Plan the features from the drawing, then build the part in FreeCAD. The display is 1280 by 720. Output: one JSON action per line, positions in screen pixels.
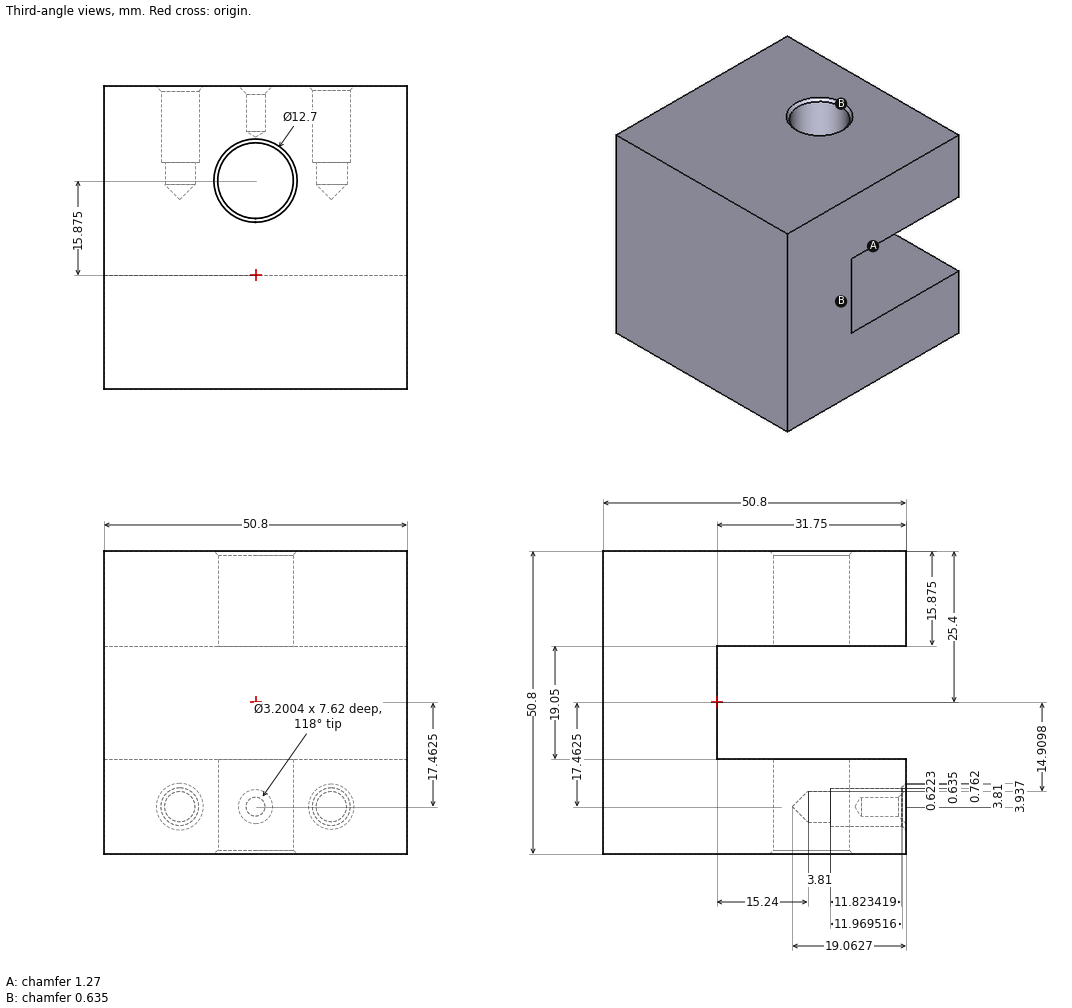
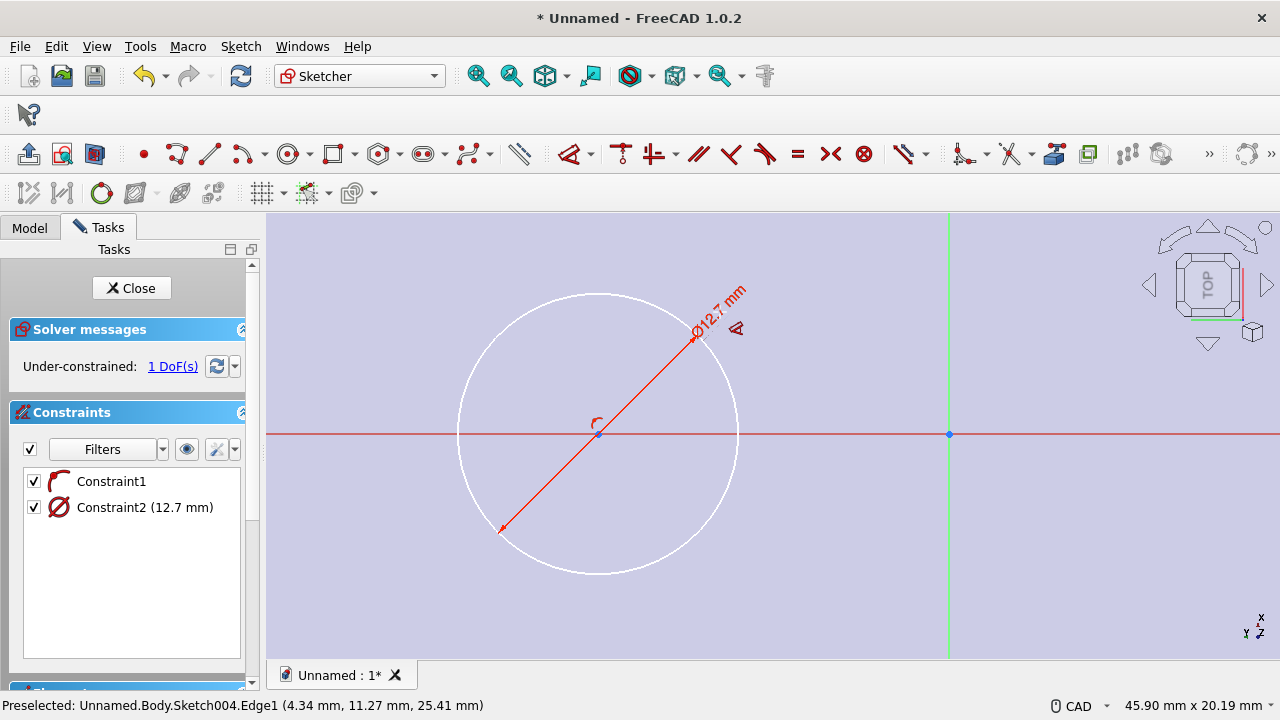
{"action": "left_click", "coordinate": [598, 434]}
{"action": "left_click", "coordinate": [774, 468]}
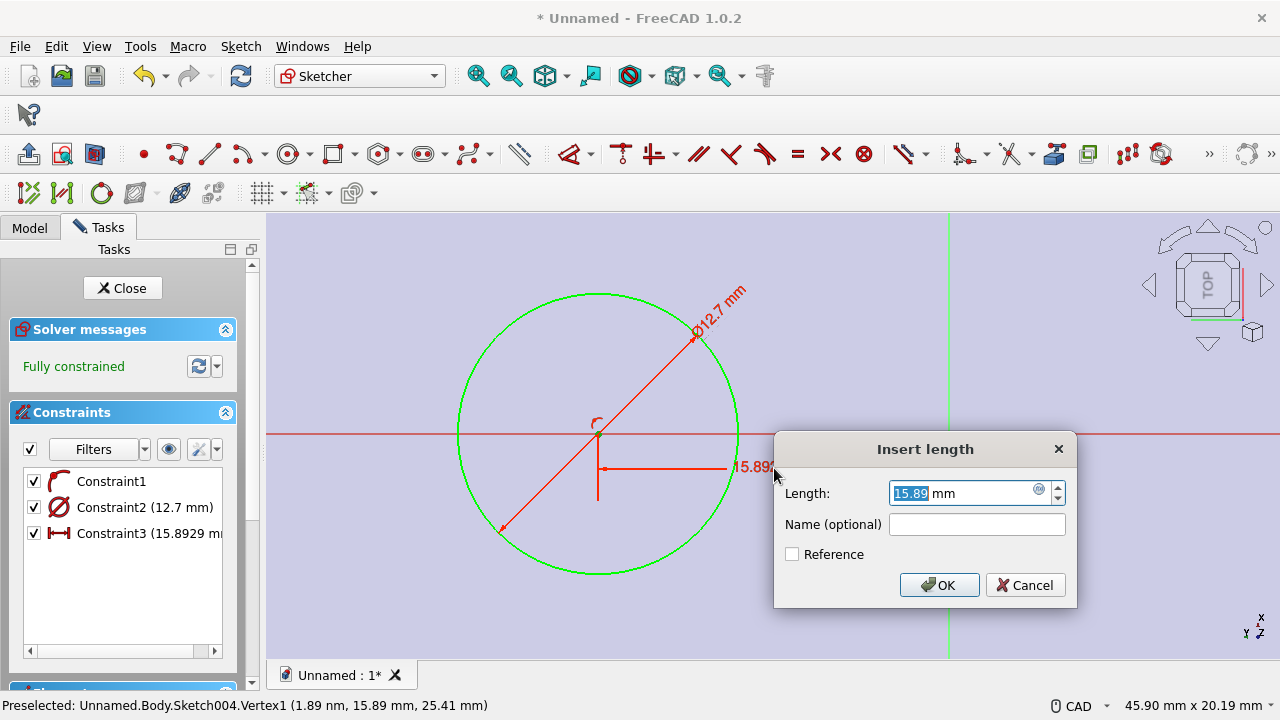
{"action": "type", "text": "15.875"}
{"action": "key", "text": "Return"}
{"action": "key", "text": "Escape"}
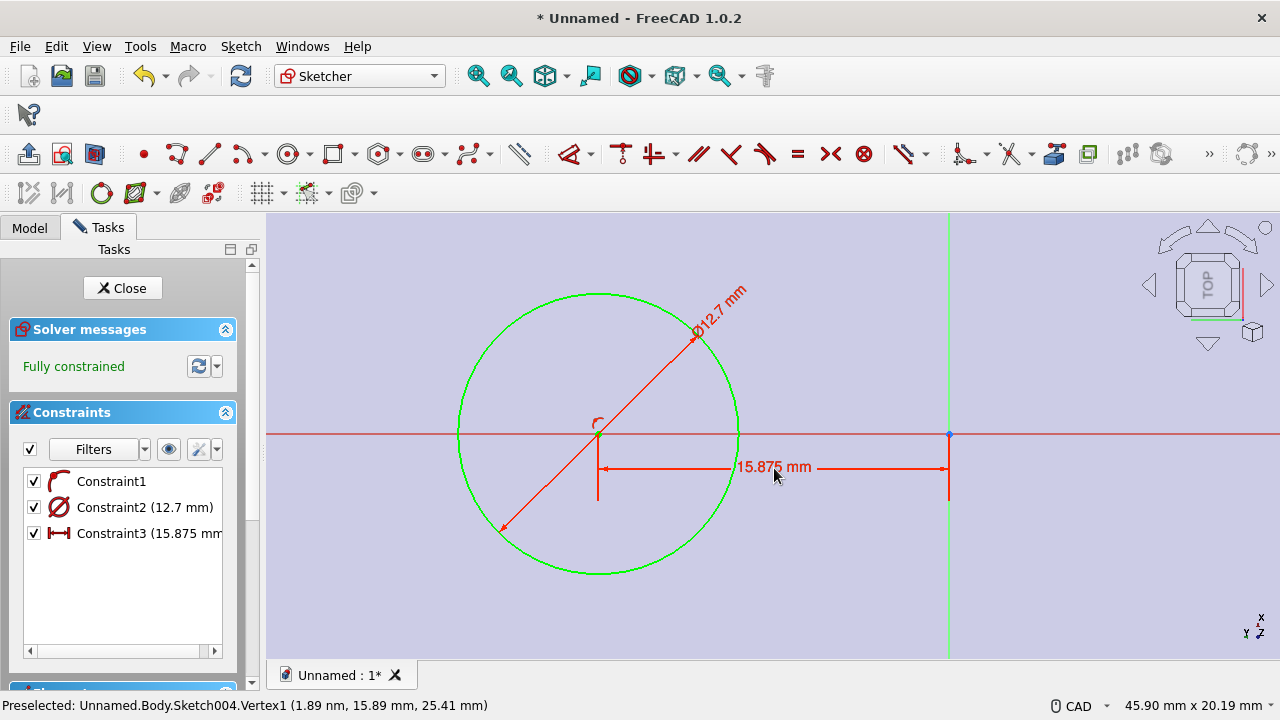
{"action": "left_click", "coordinate": [123, 288]}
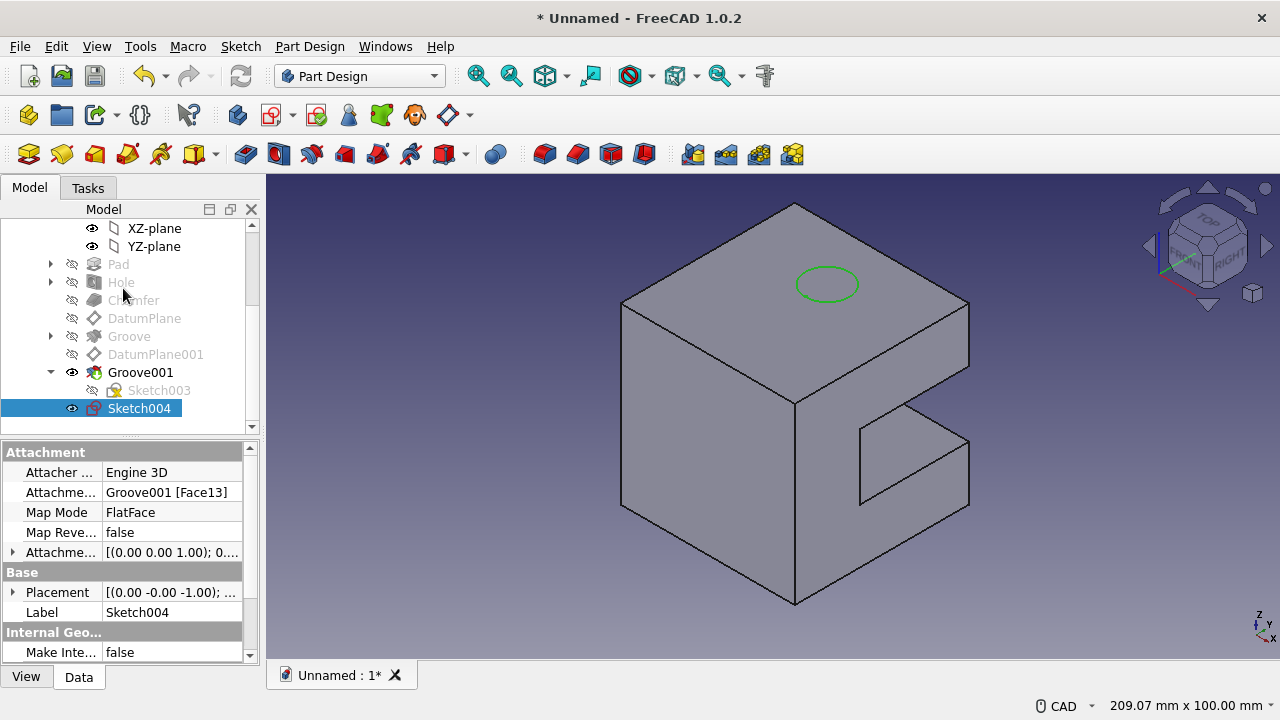
{"action": "left_click", "coordinate": [246, 154]}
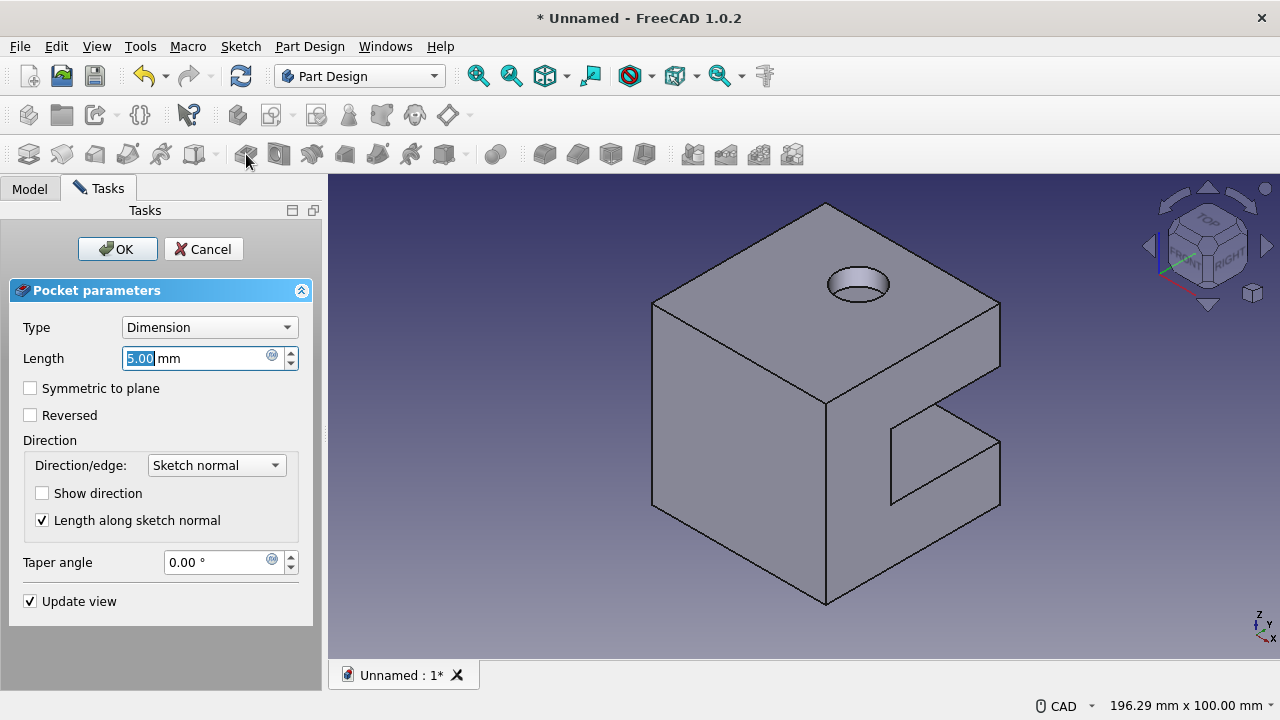
{"action": "left_click", "coordinate": [210, 328]}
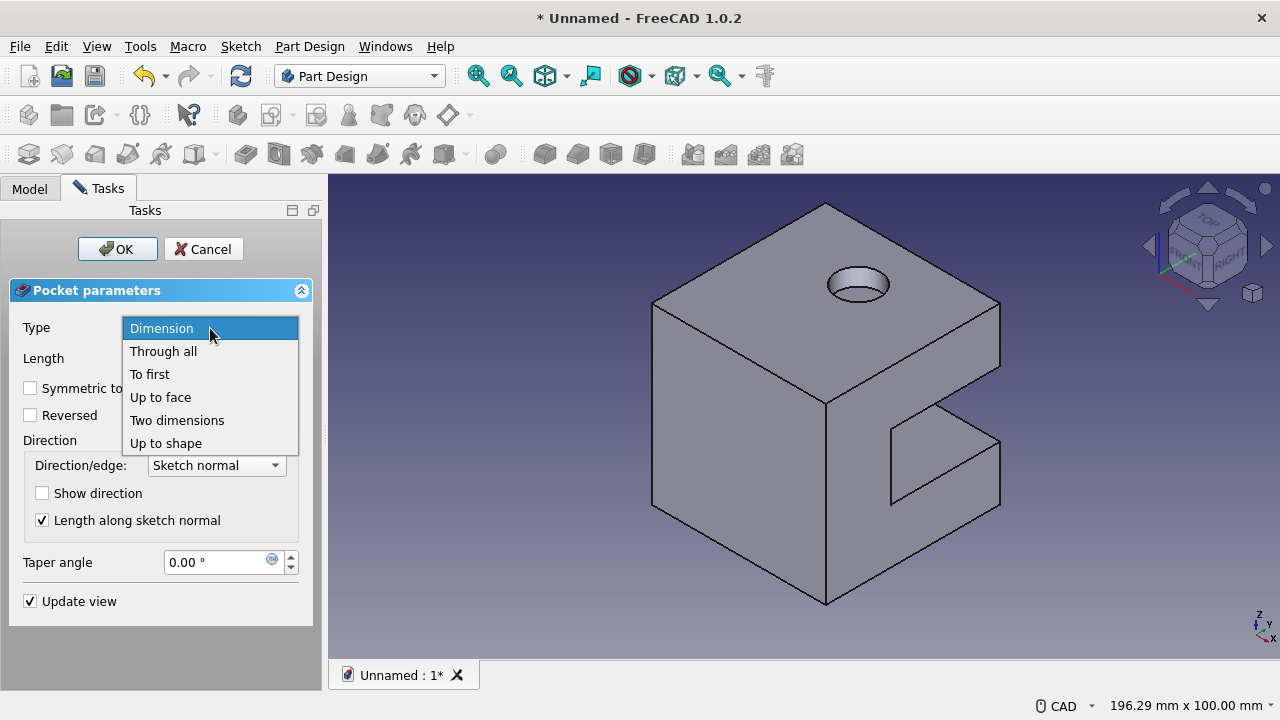
{"action": "left_click", "coordinate": [208, 352]}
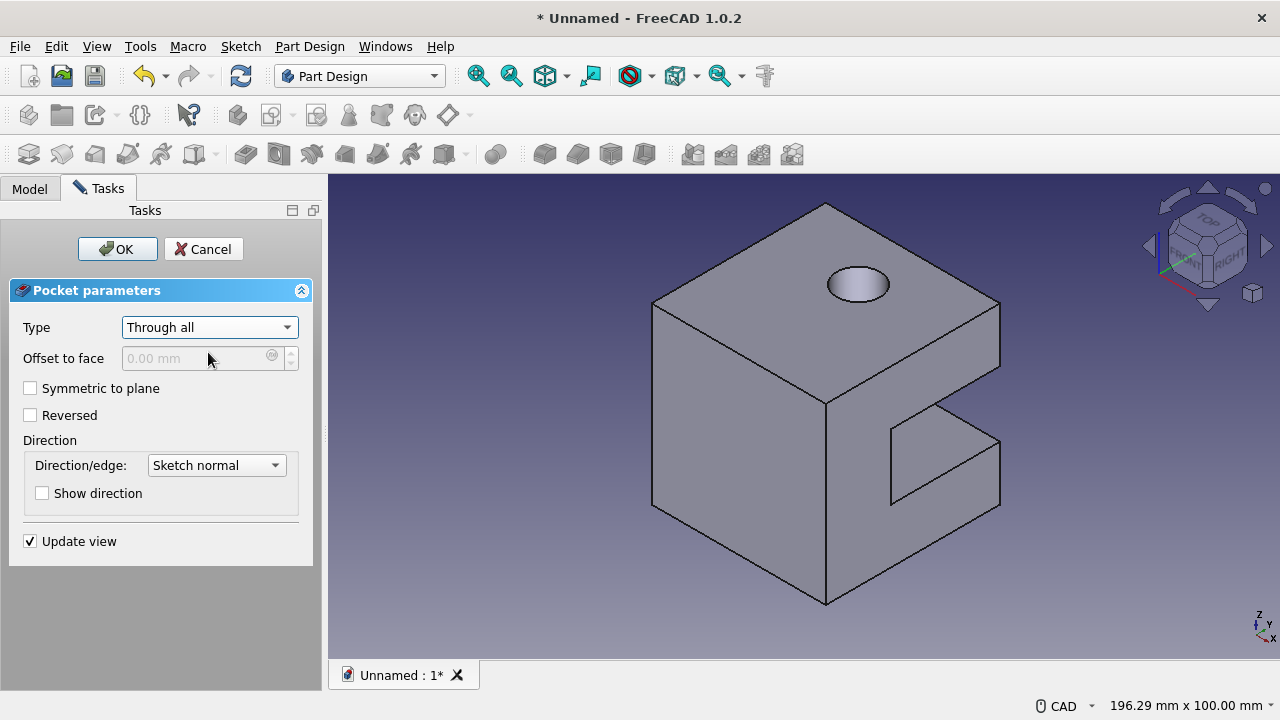
{"action": "left_click", "coordinate": [118, 249]}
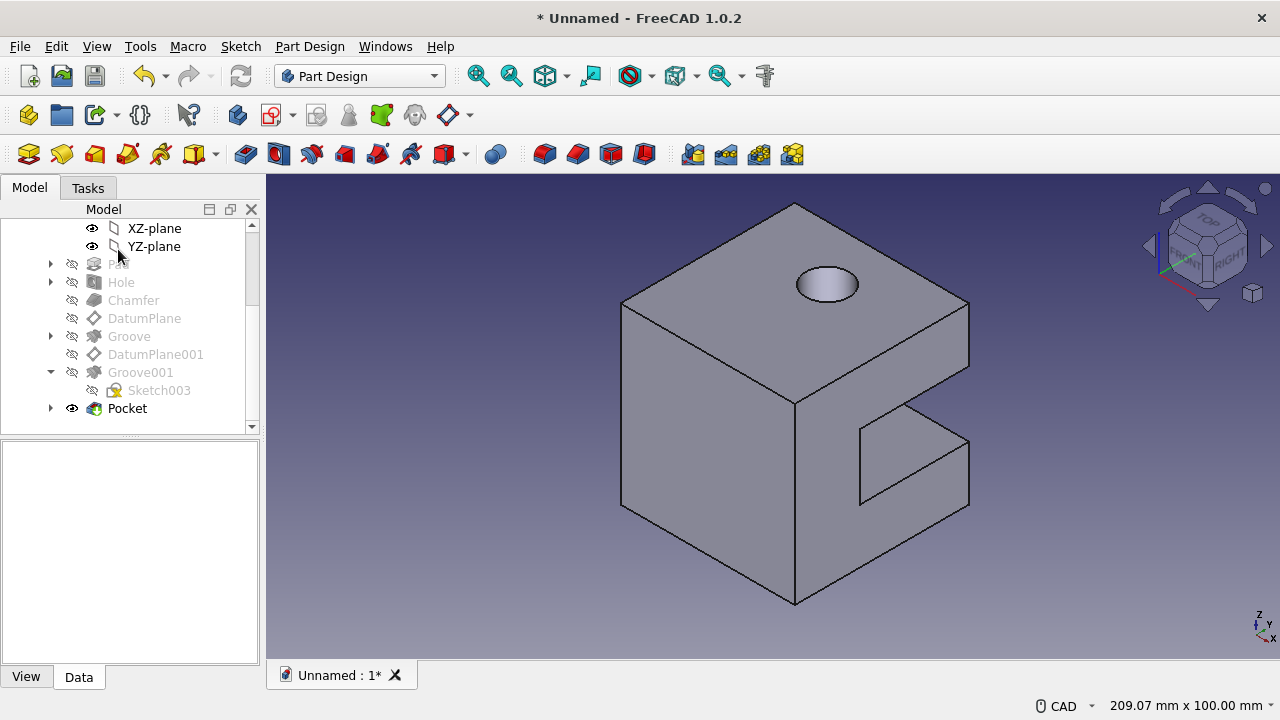
{"action": "left_click", "coordinate": [849, 271]}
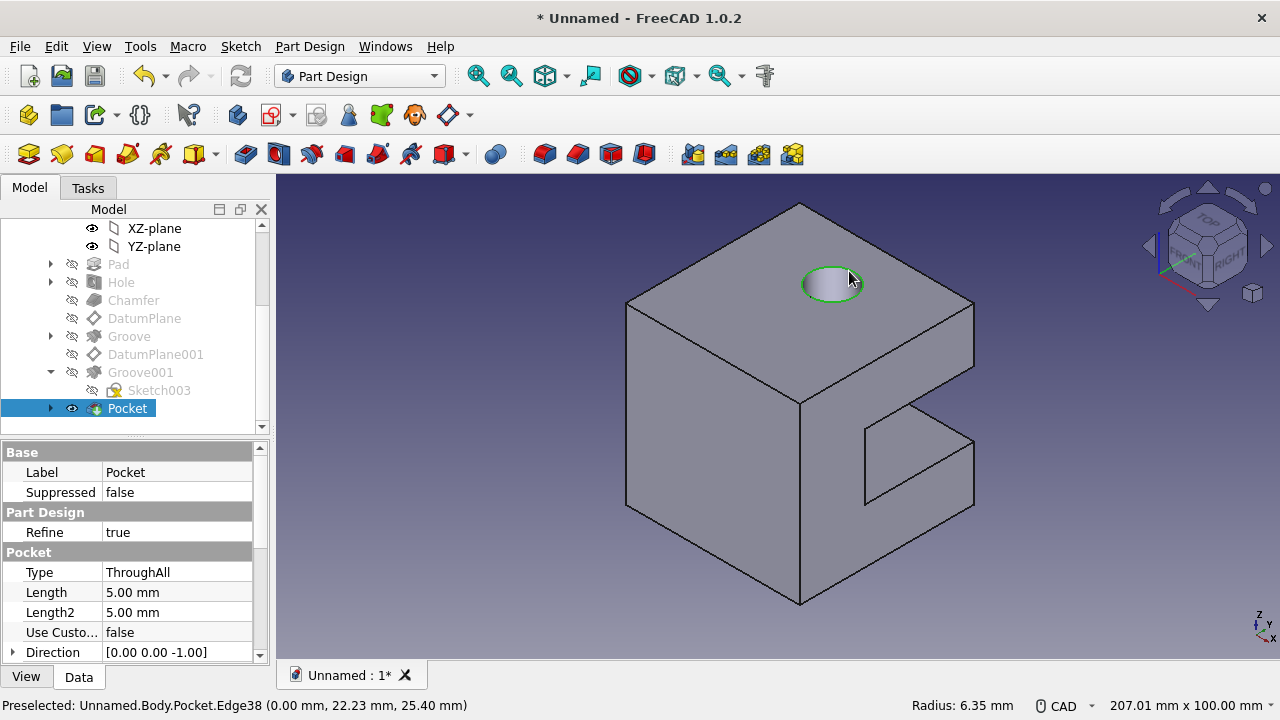
{"action": "key", "text": "2"}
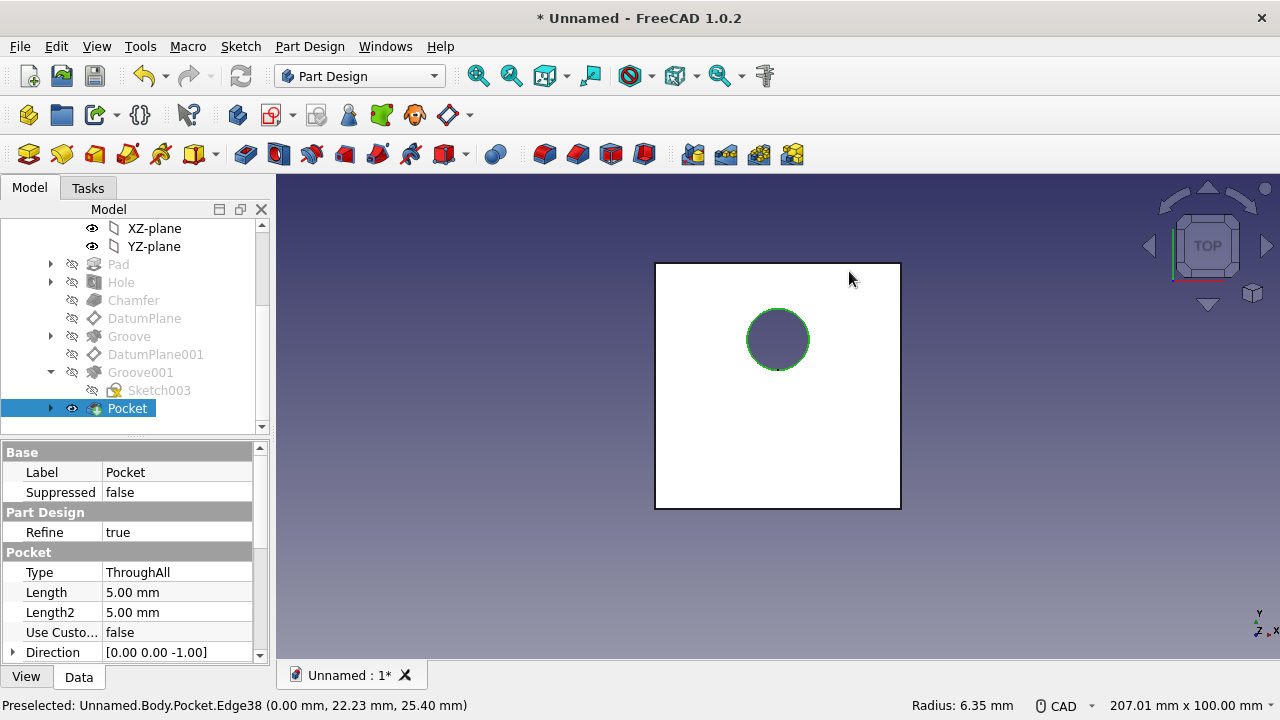
{"action": "key", "text": "0"}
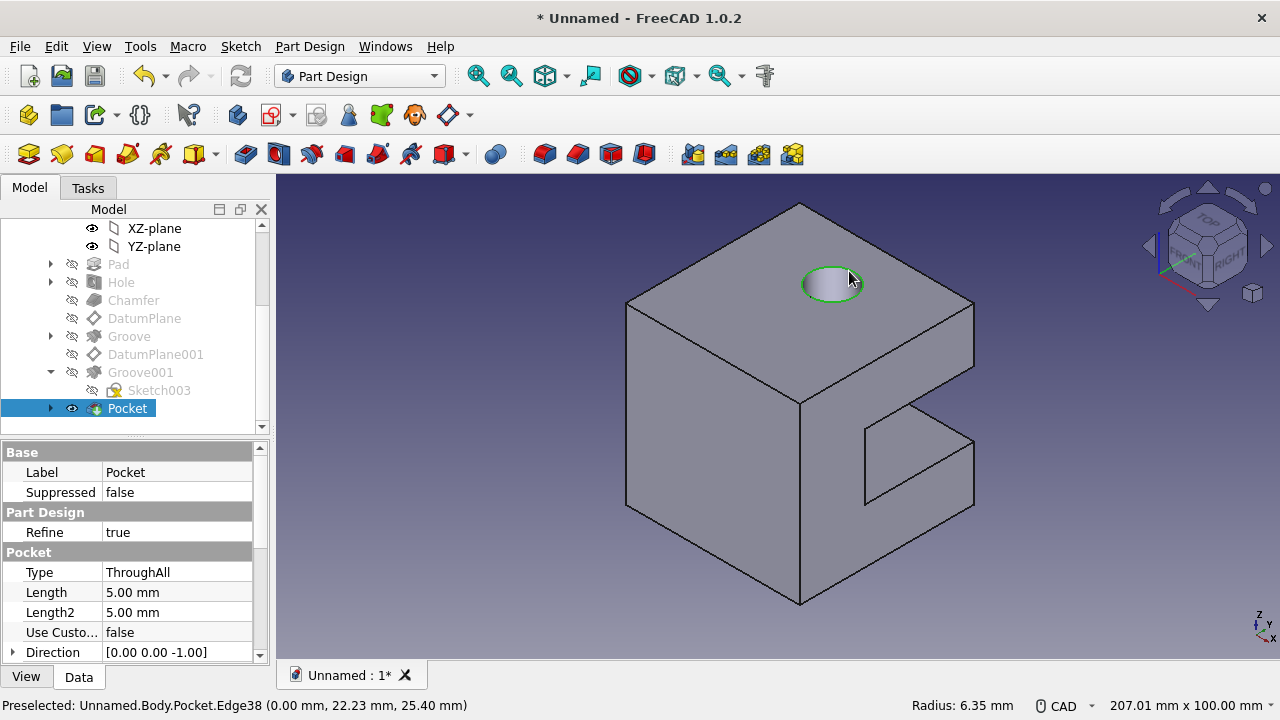
{"action": "key", "text": "1"}